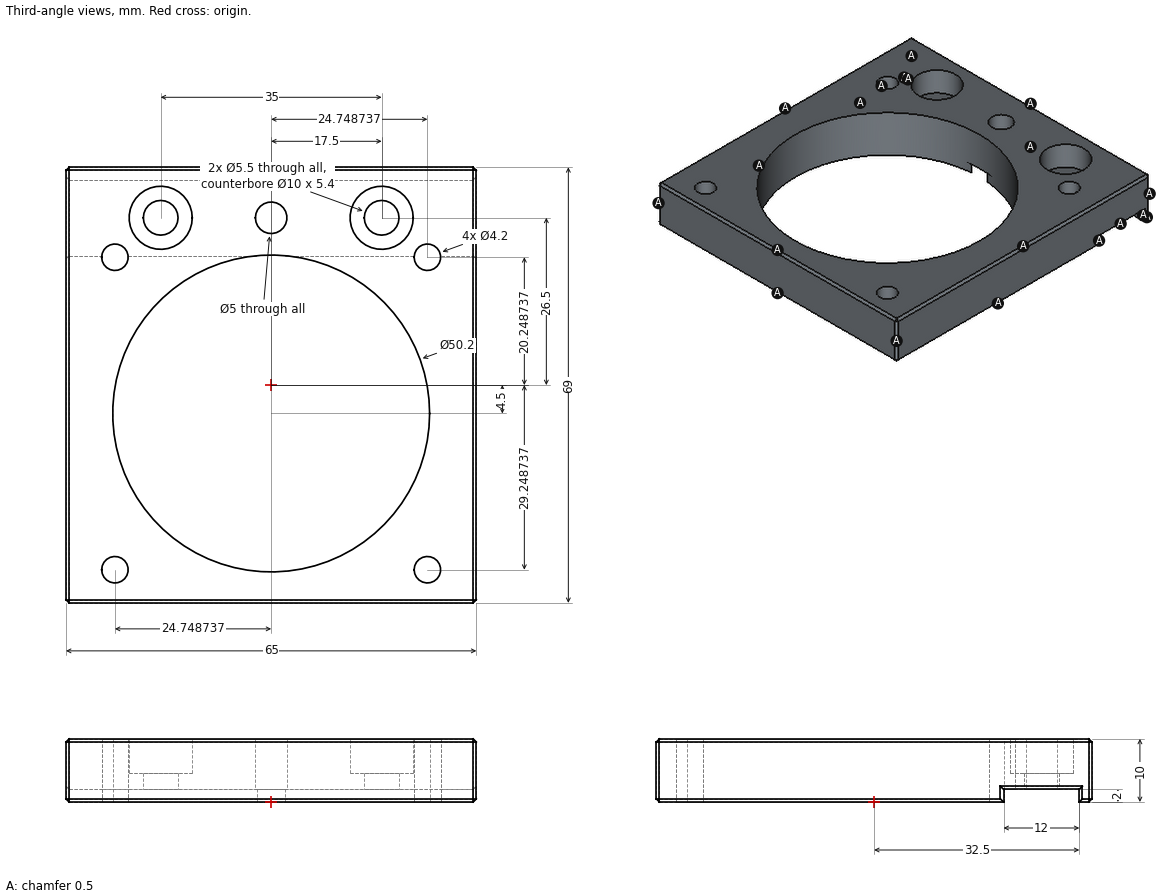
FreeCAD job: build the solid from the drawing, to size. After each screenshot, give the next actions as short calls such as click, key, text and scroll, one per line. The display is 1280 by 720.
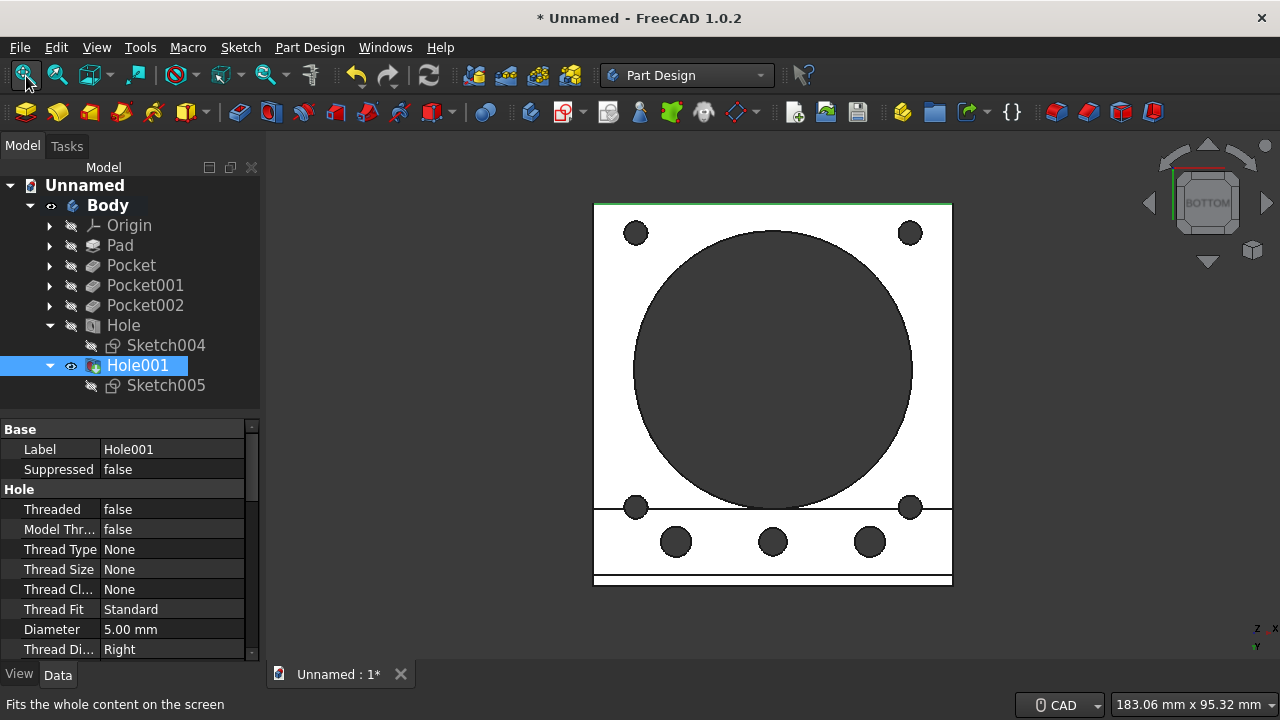
click(773, 585, ctrl)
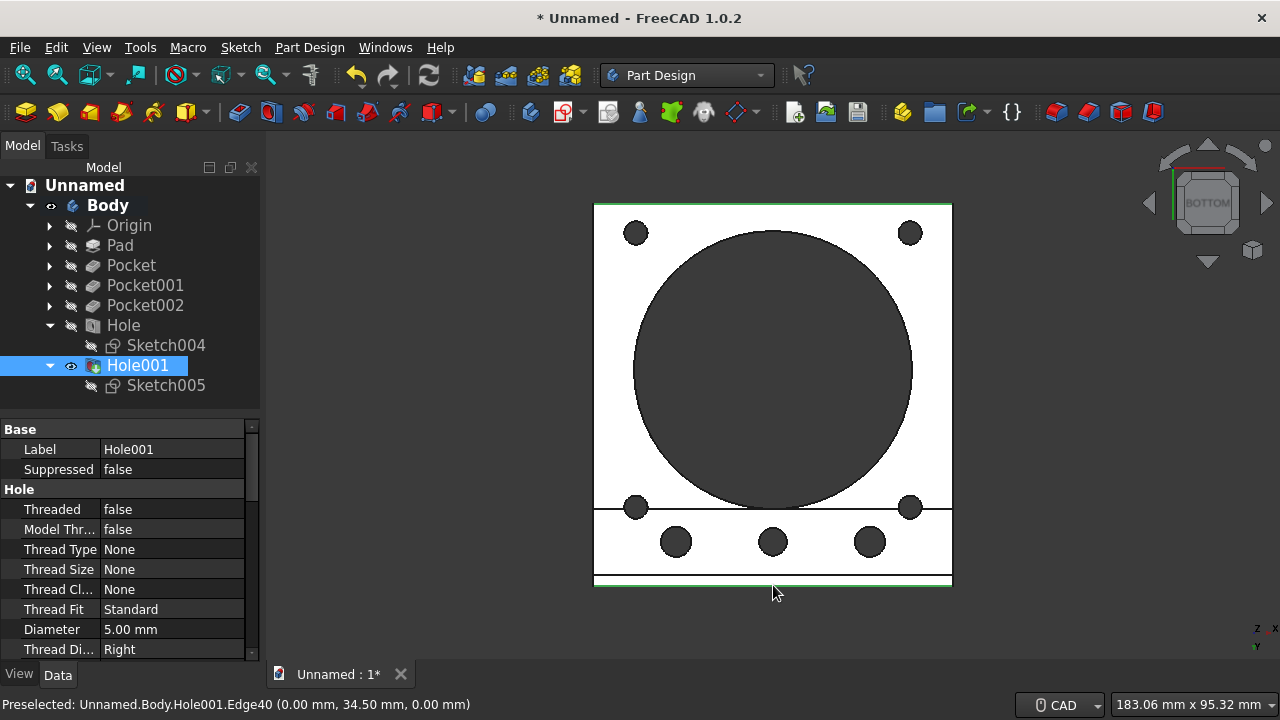
key(4)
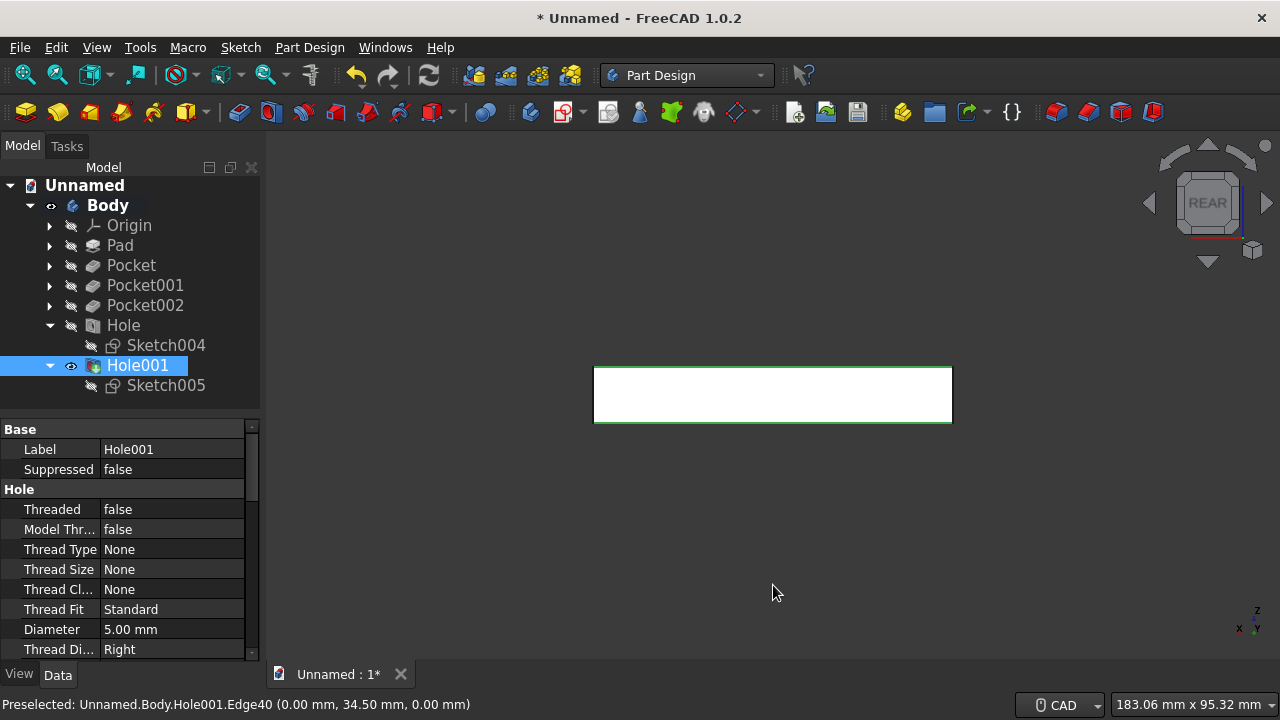
click(26, 76)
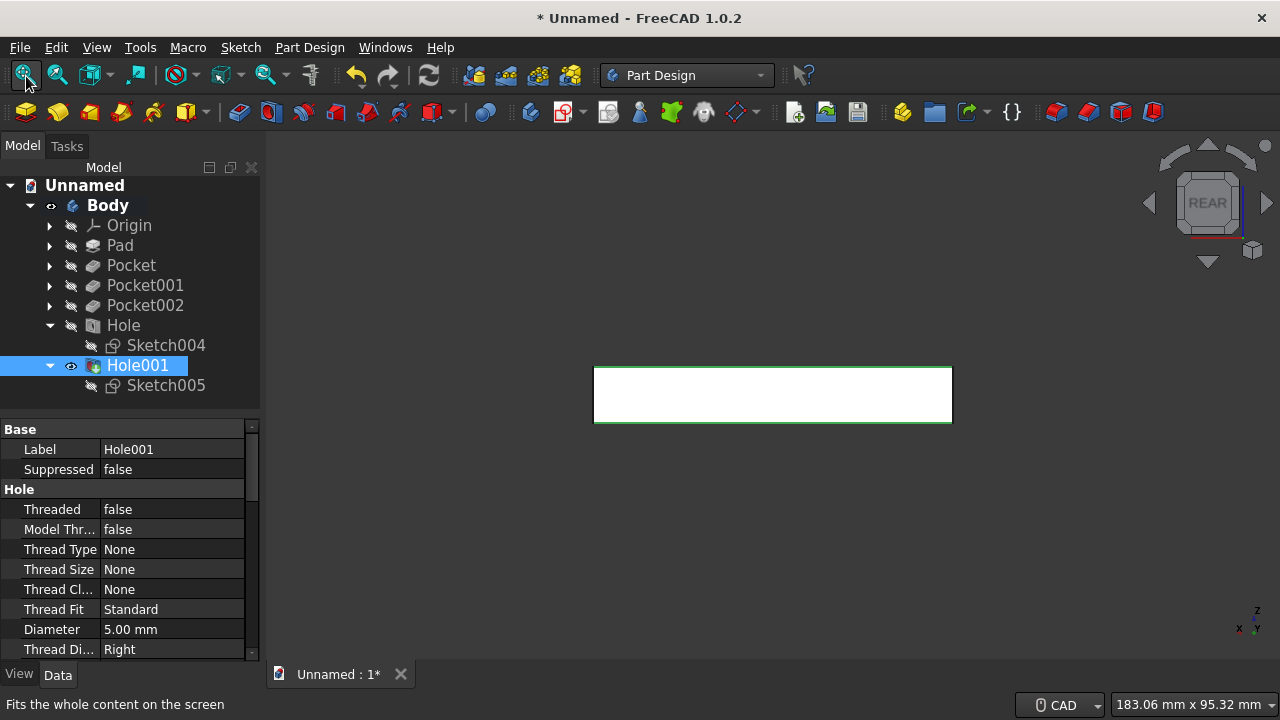
key(6)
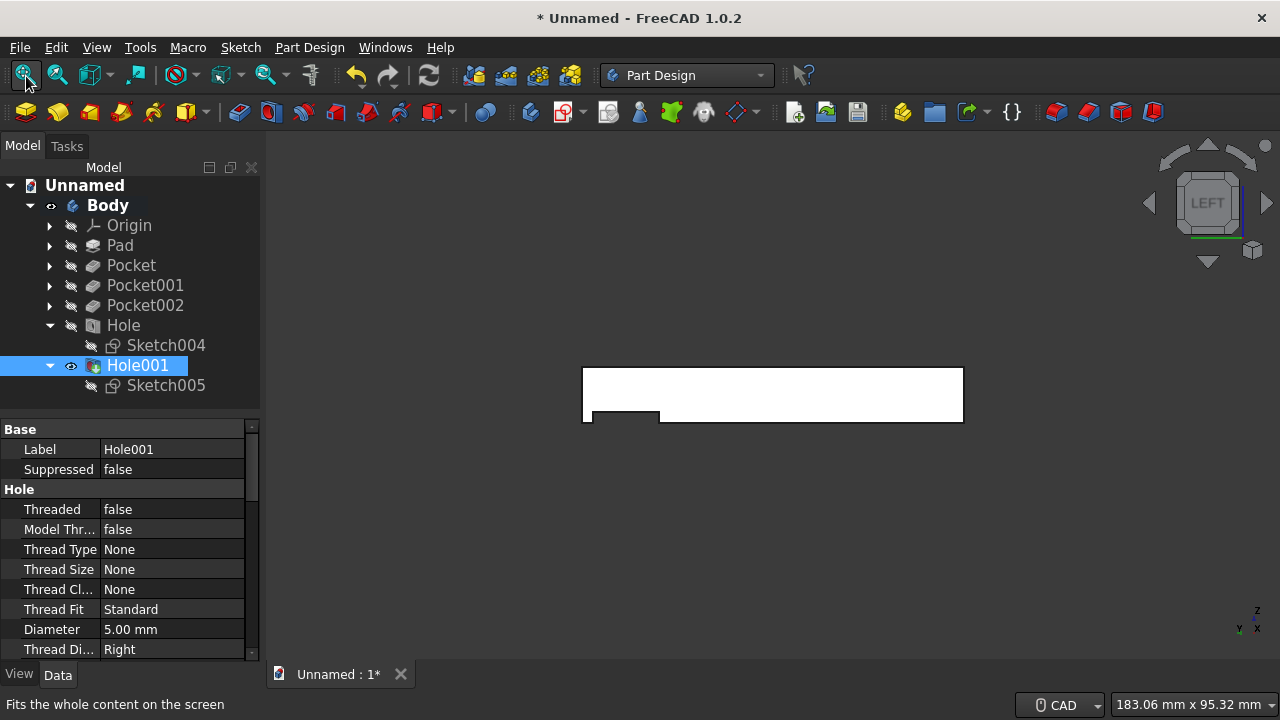
click(26, 76)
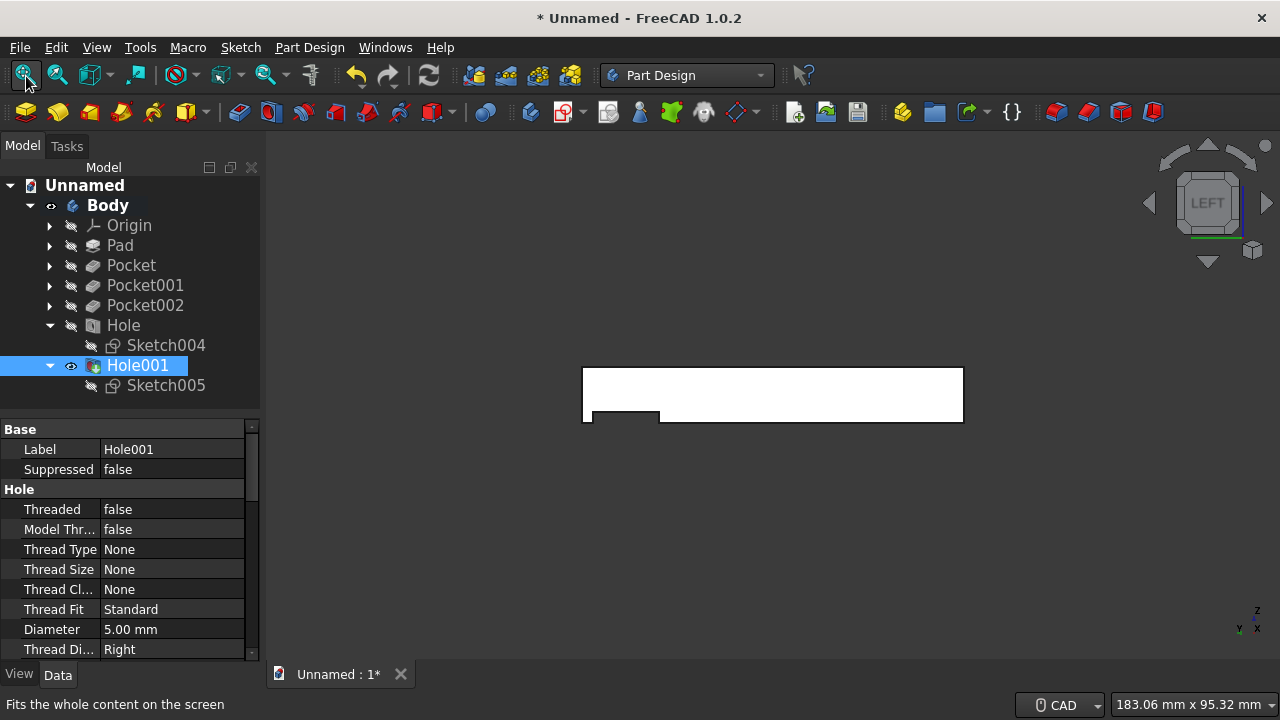
click(718, 394, ctrl)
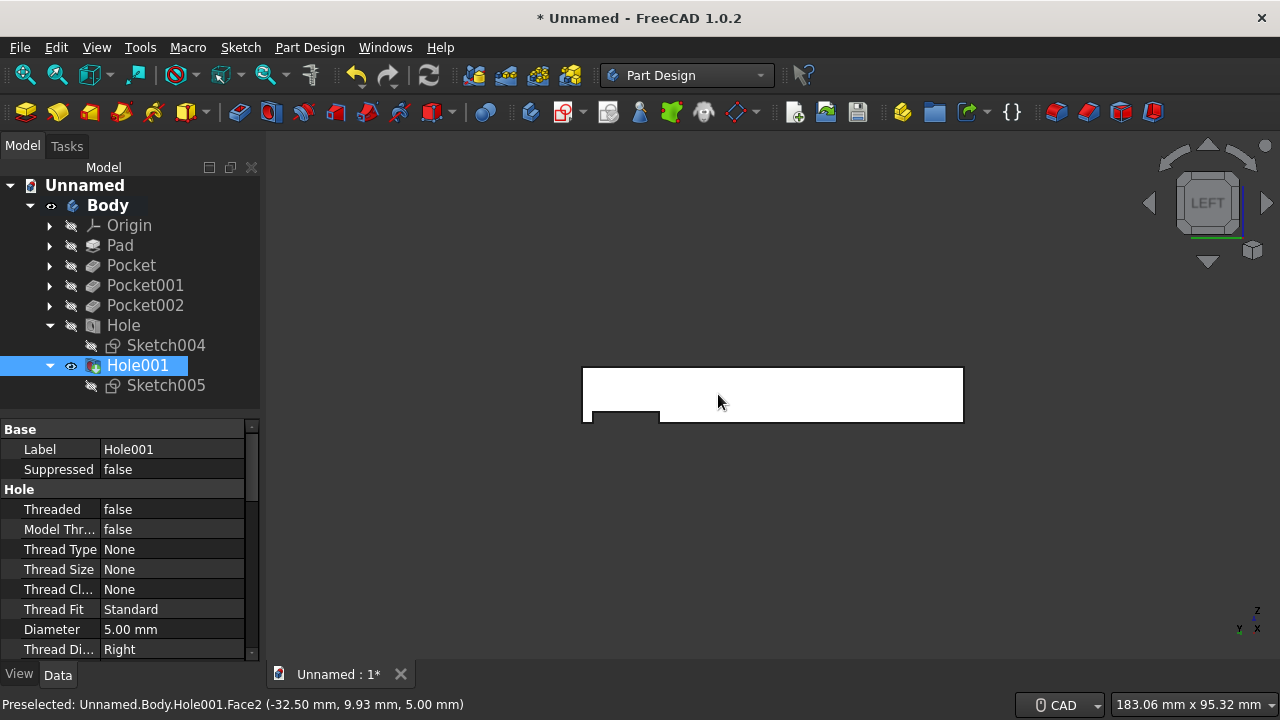
click(1090, 112)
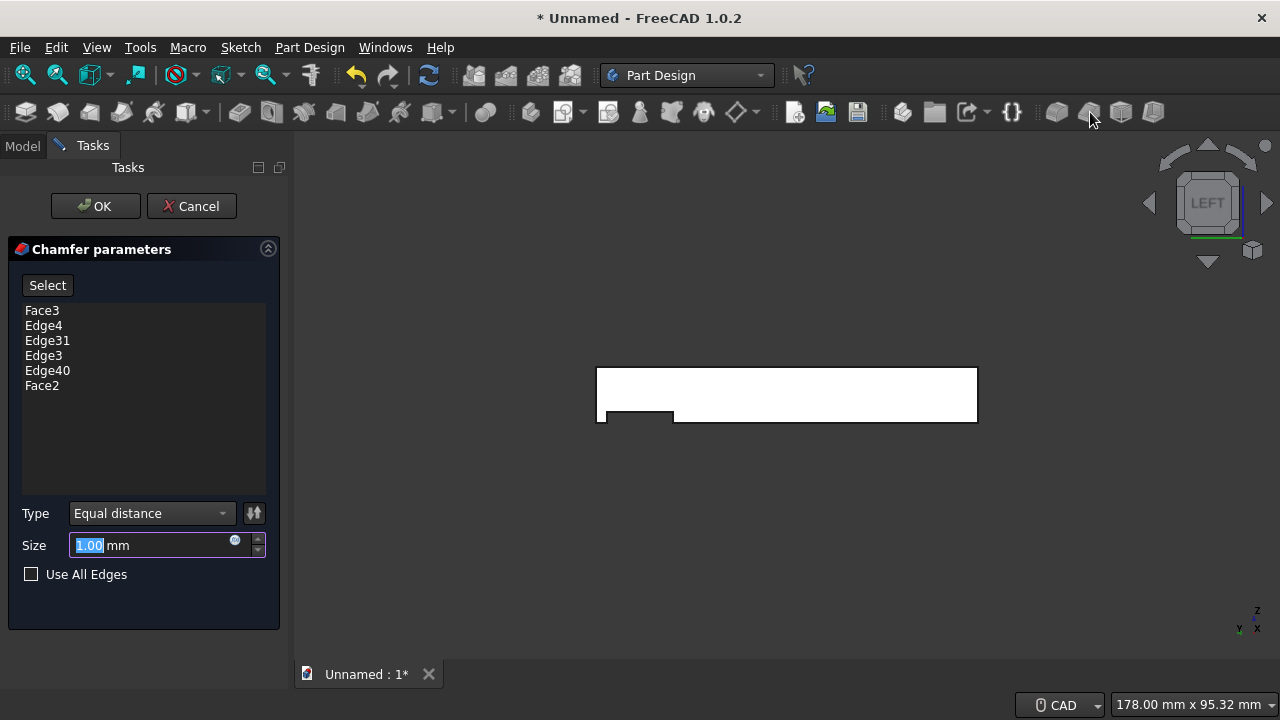
text(0.5)
key(Tab)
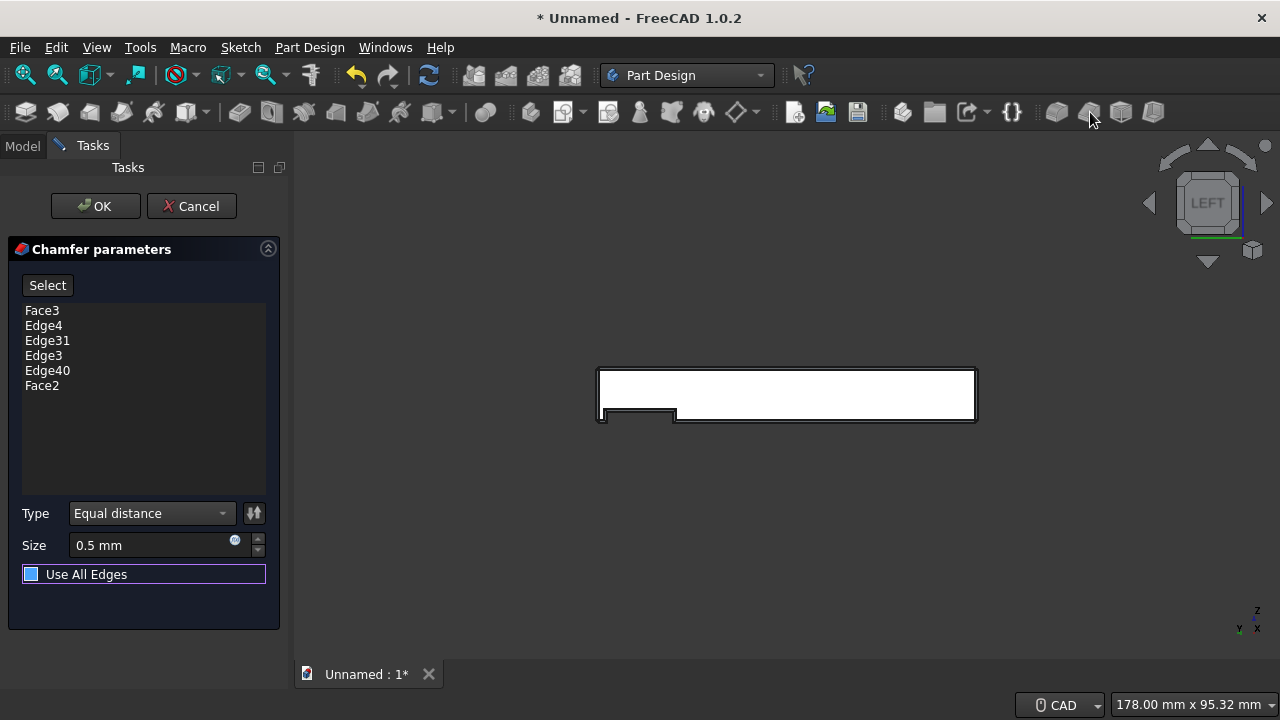
click(96, 206)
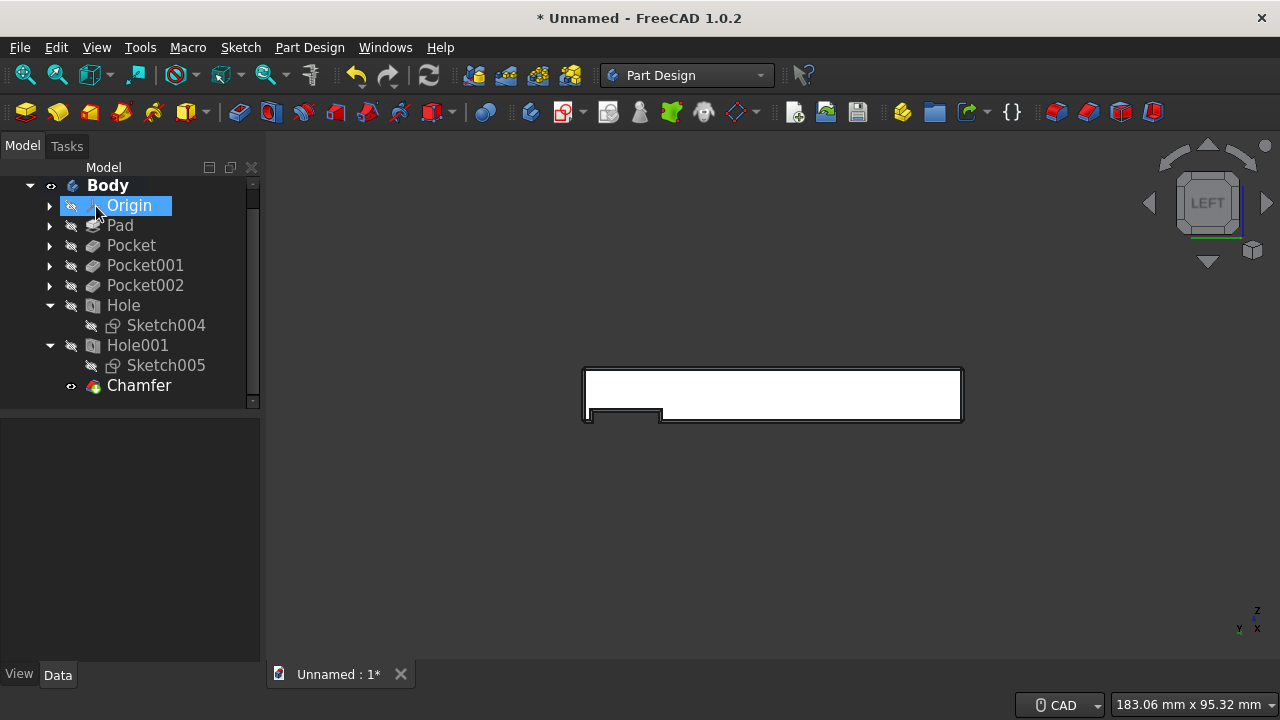
key(0)